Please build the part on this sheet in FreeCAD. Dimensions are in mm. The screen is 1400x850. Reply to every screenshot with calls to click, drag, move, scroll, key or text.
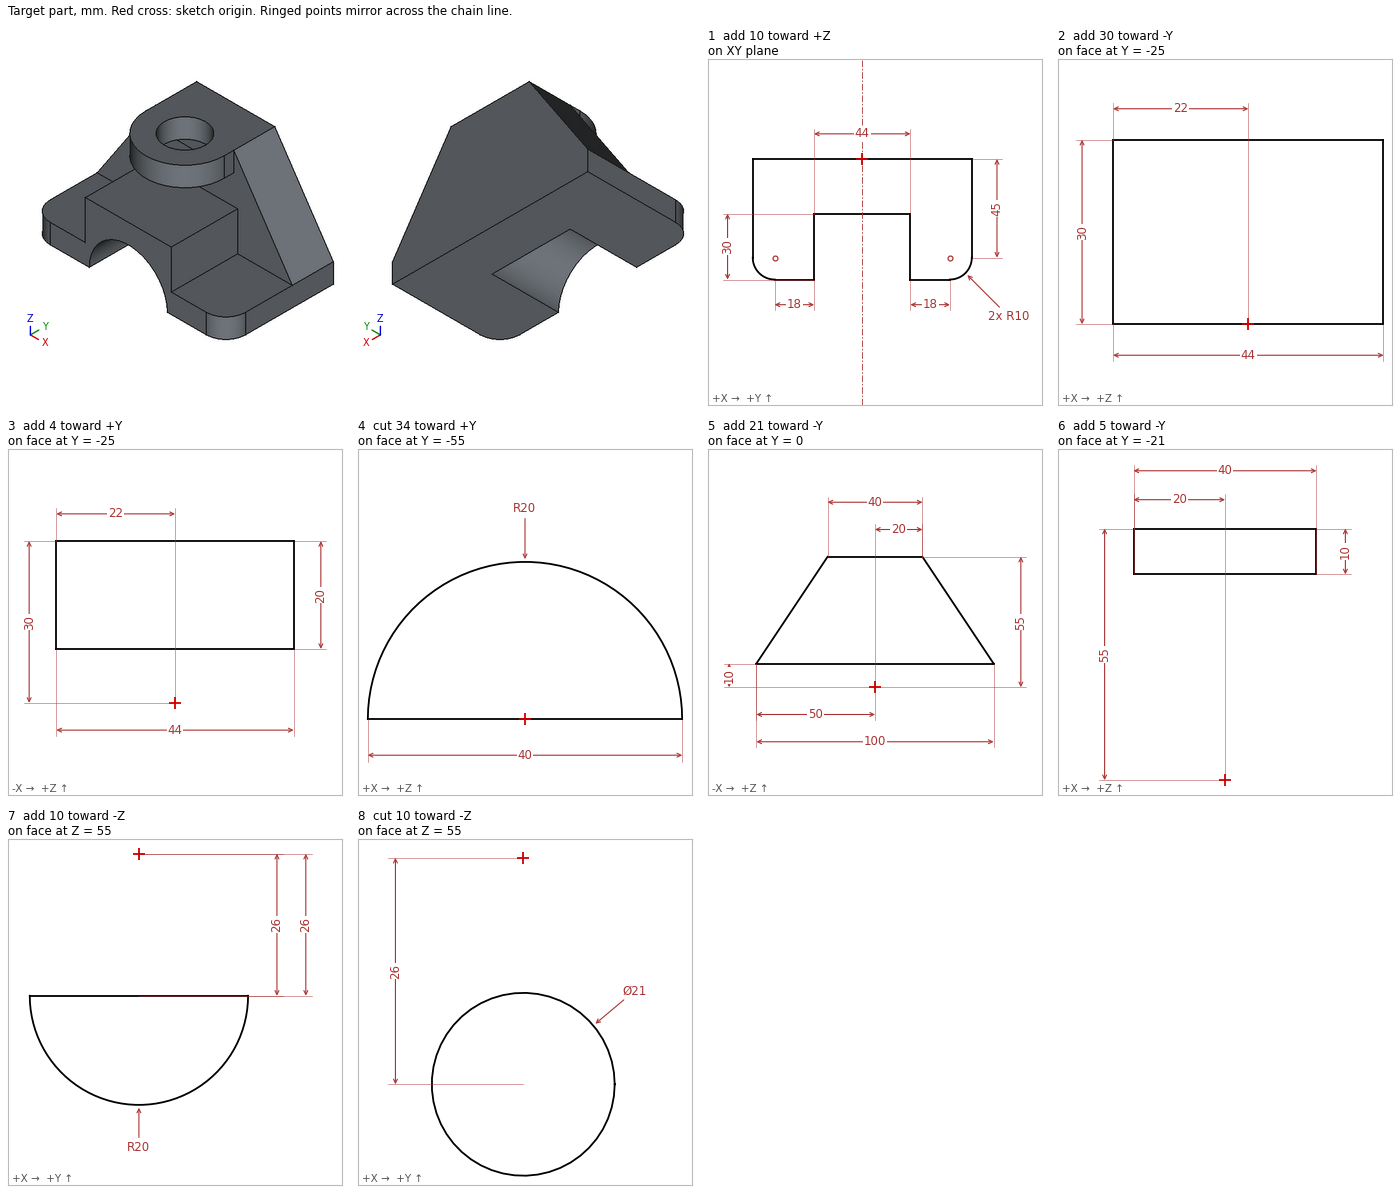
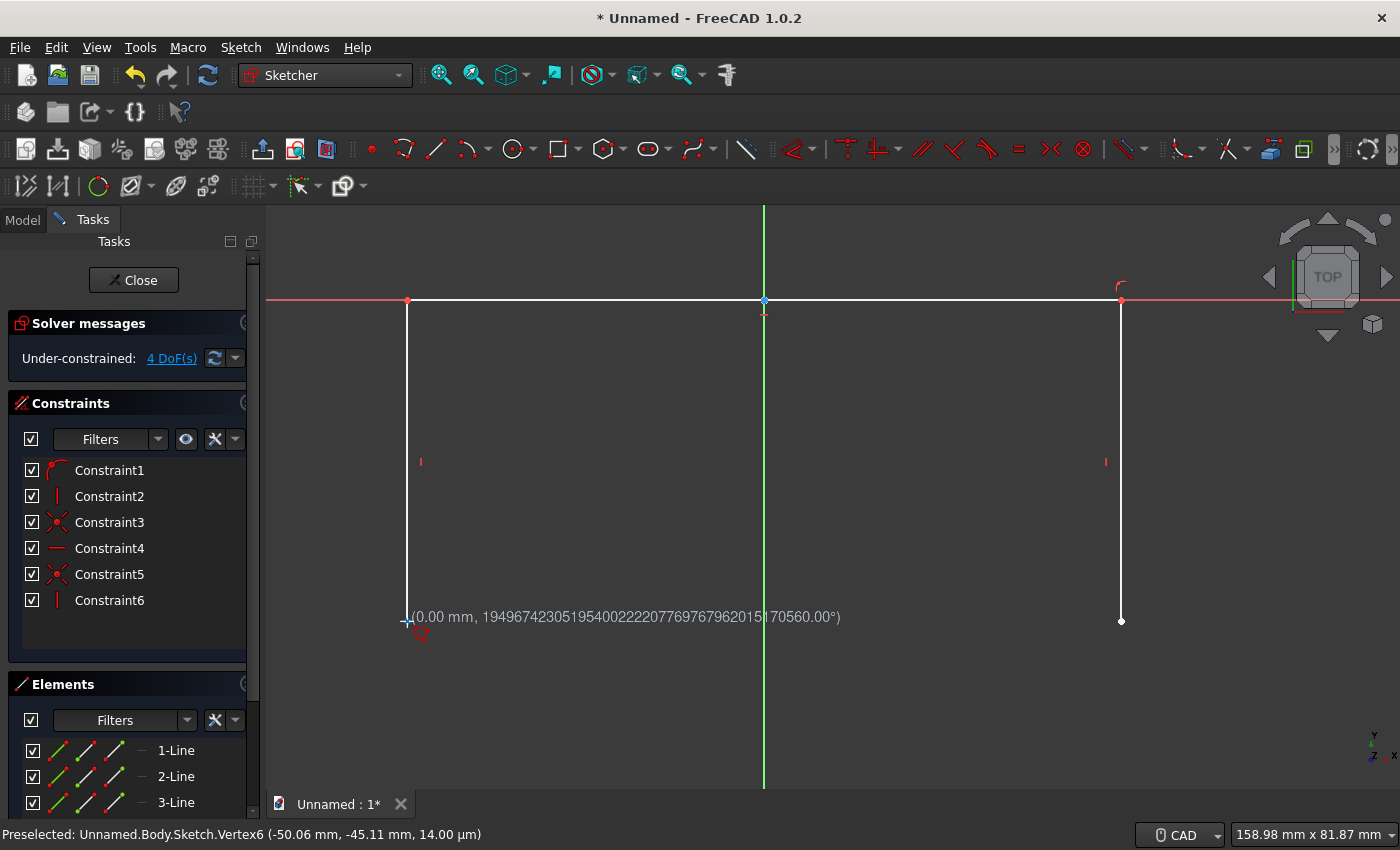
click(479, 693)
click(607, 693)
click(607, 479)
click(921, 479)
click(921, 693)
click(1049, 693)
right_click(1049, 693)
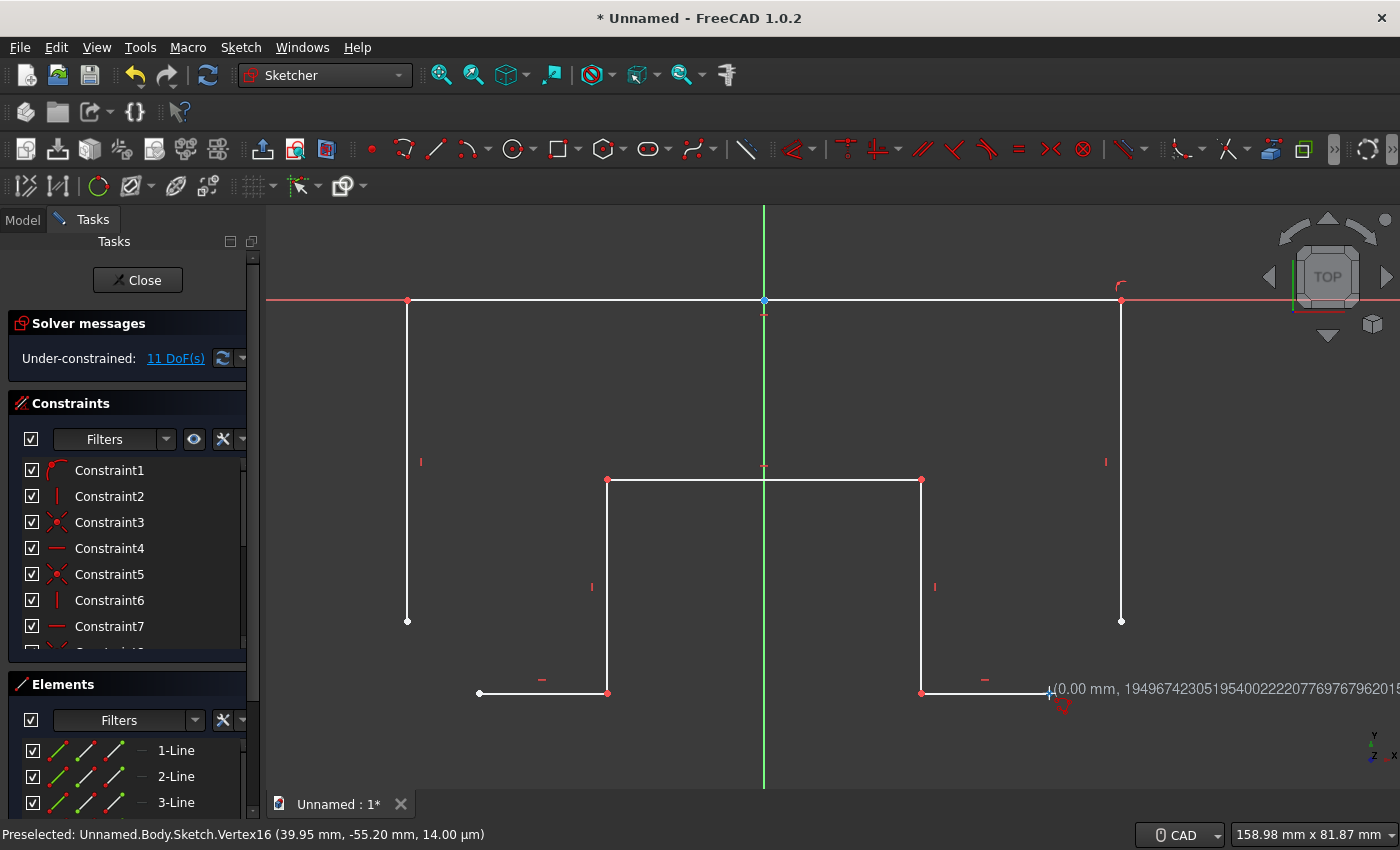
click(490, 150)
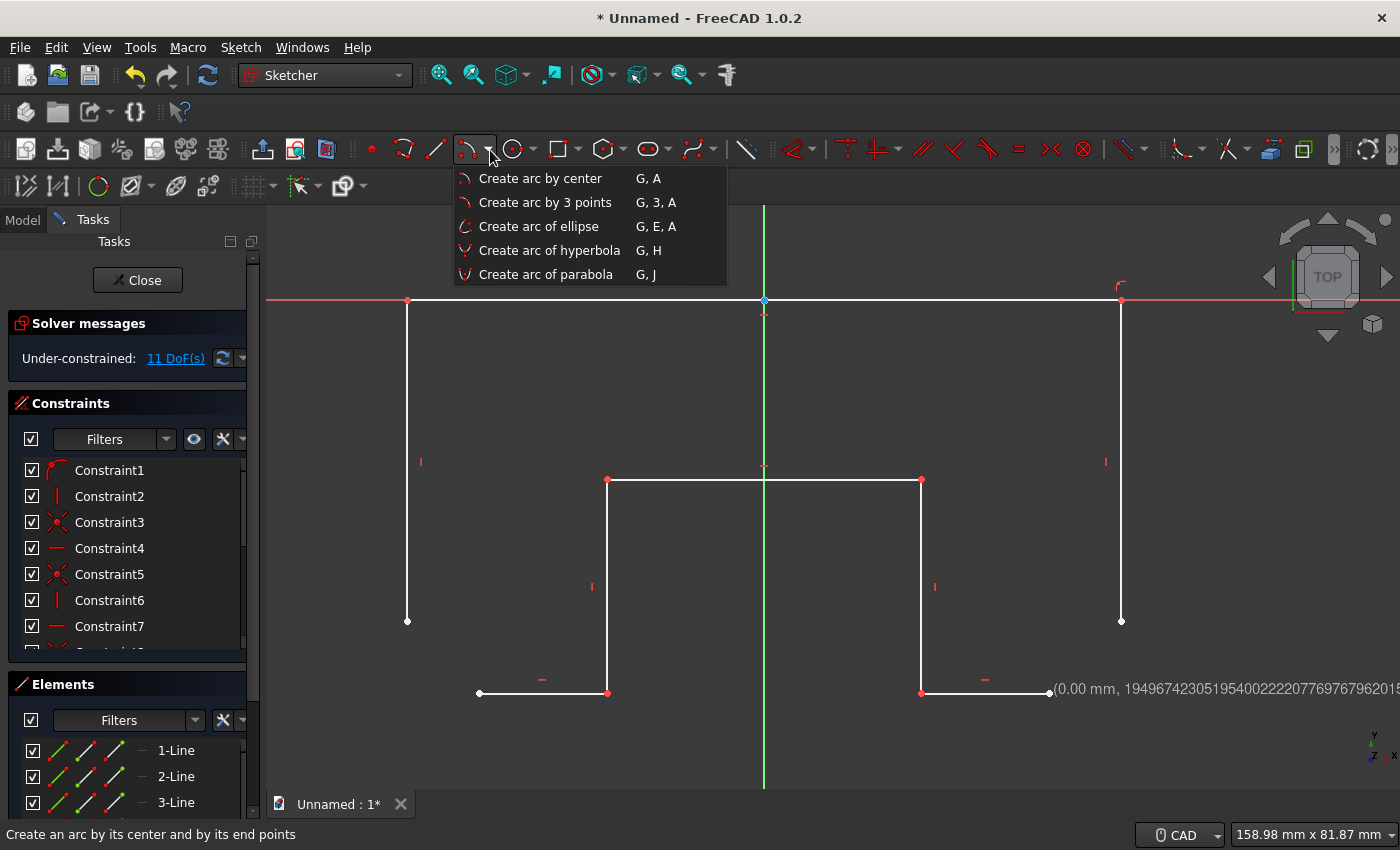
click(590, 202)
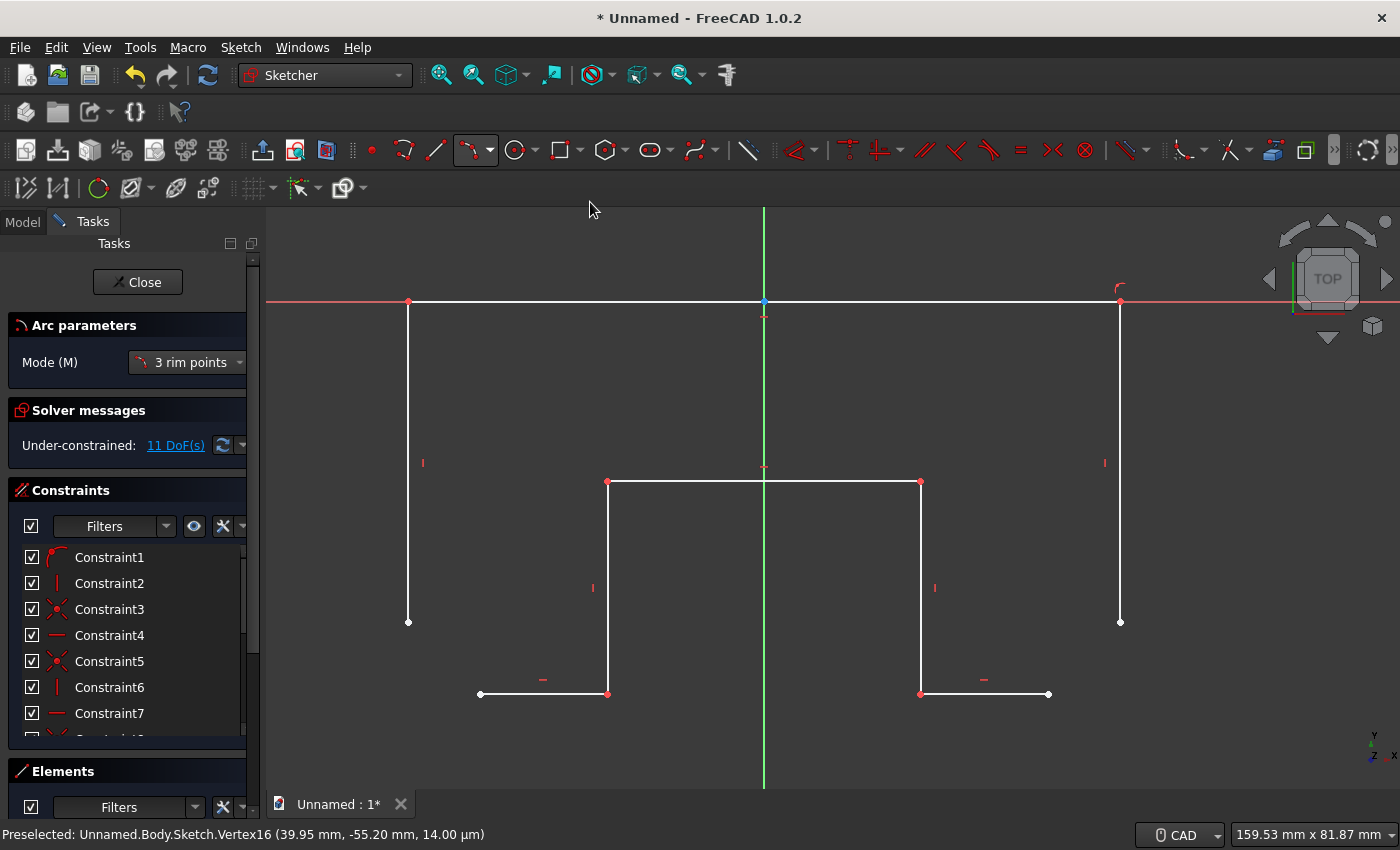
click(408, 623)
click(480, 694)
click(430, 672)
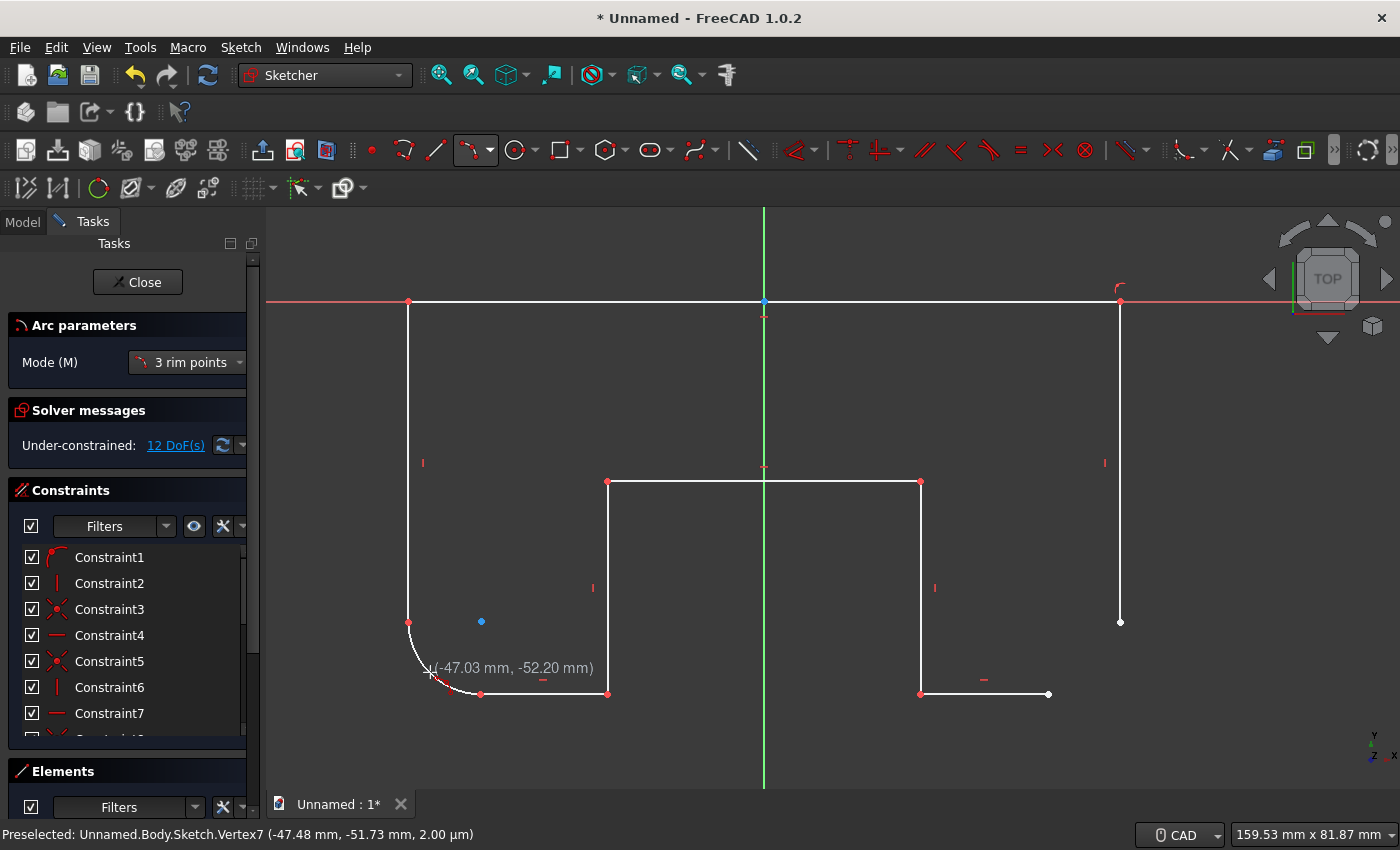
click(1048, 694)
click(1120, 623)
click(1099, 672)
key(Escape)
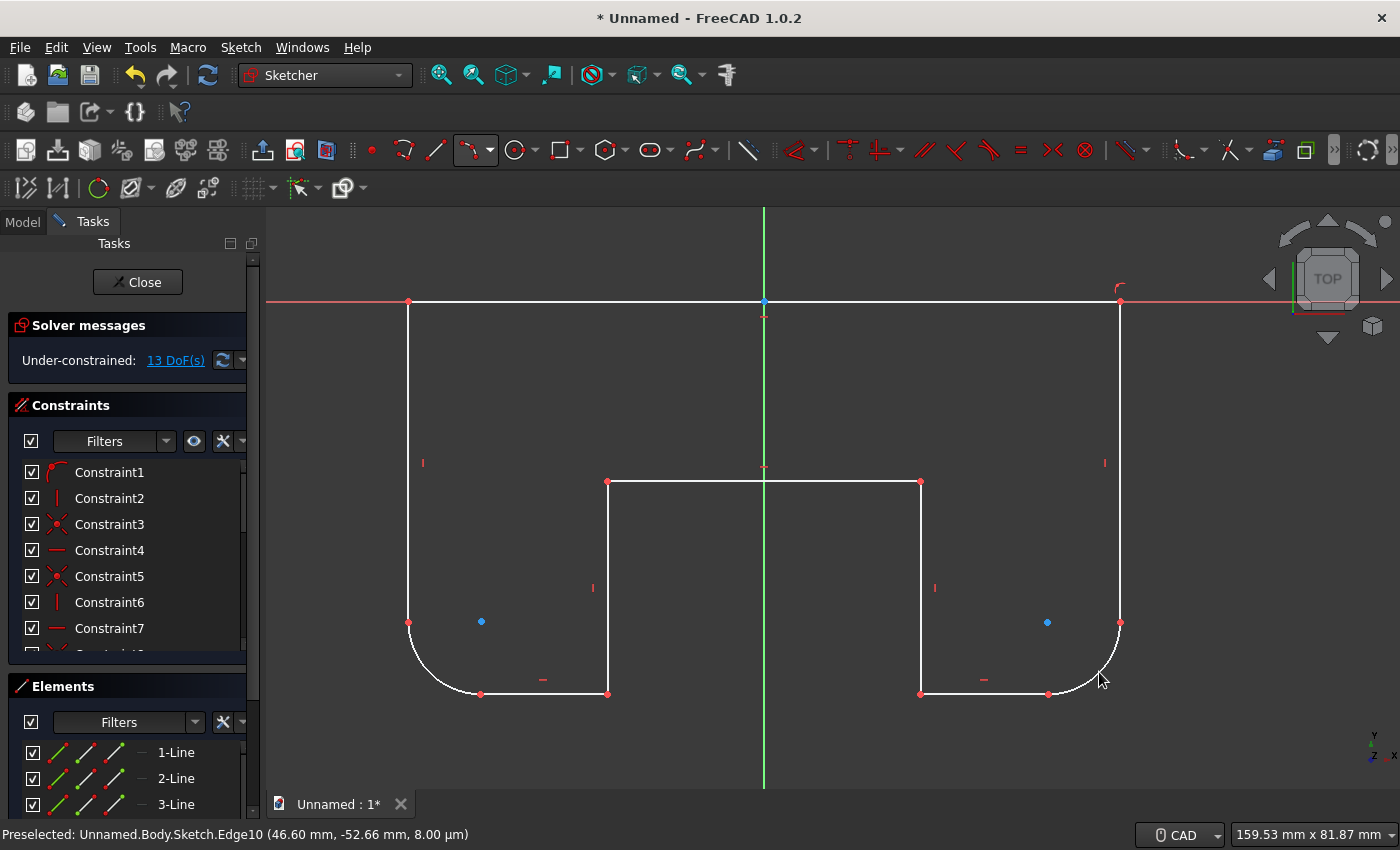
click(1120, 526)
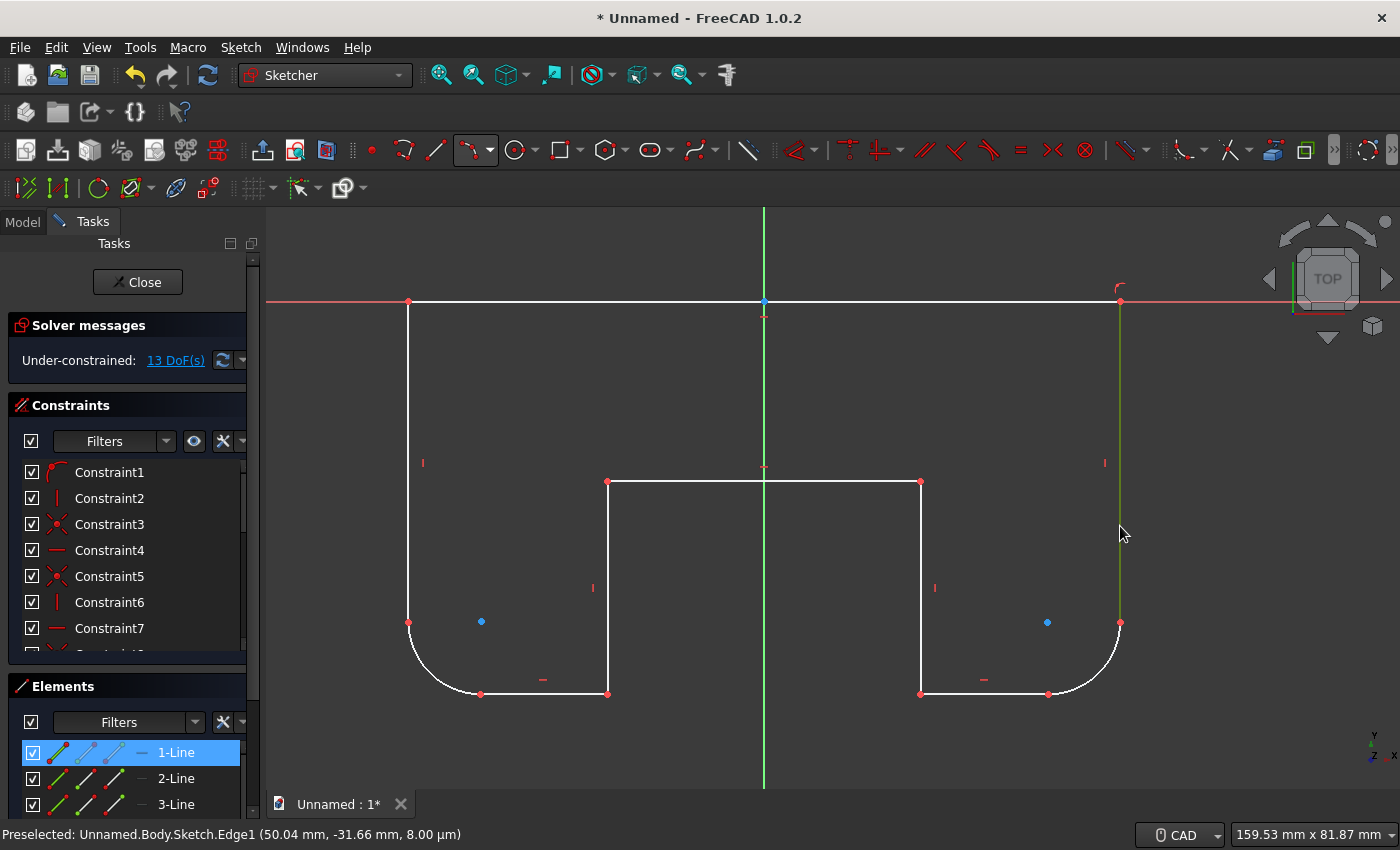
click(1081, 686)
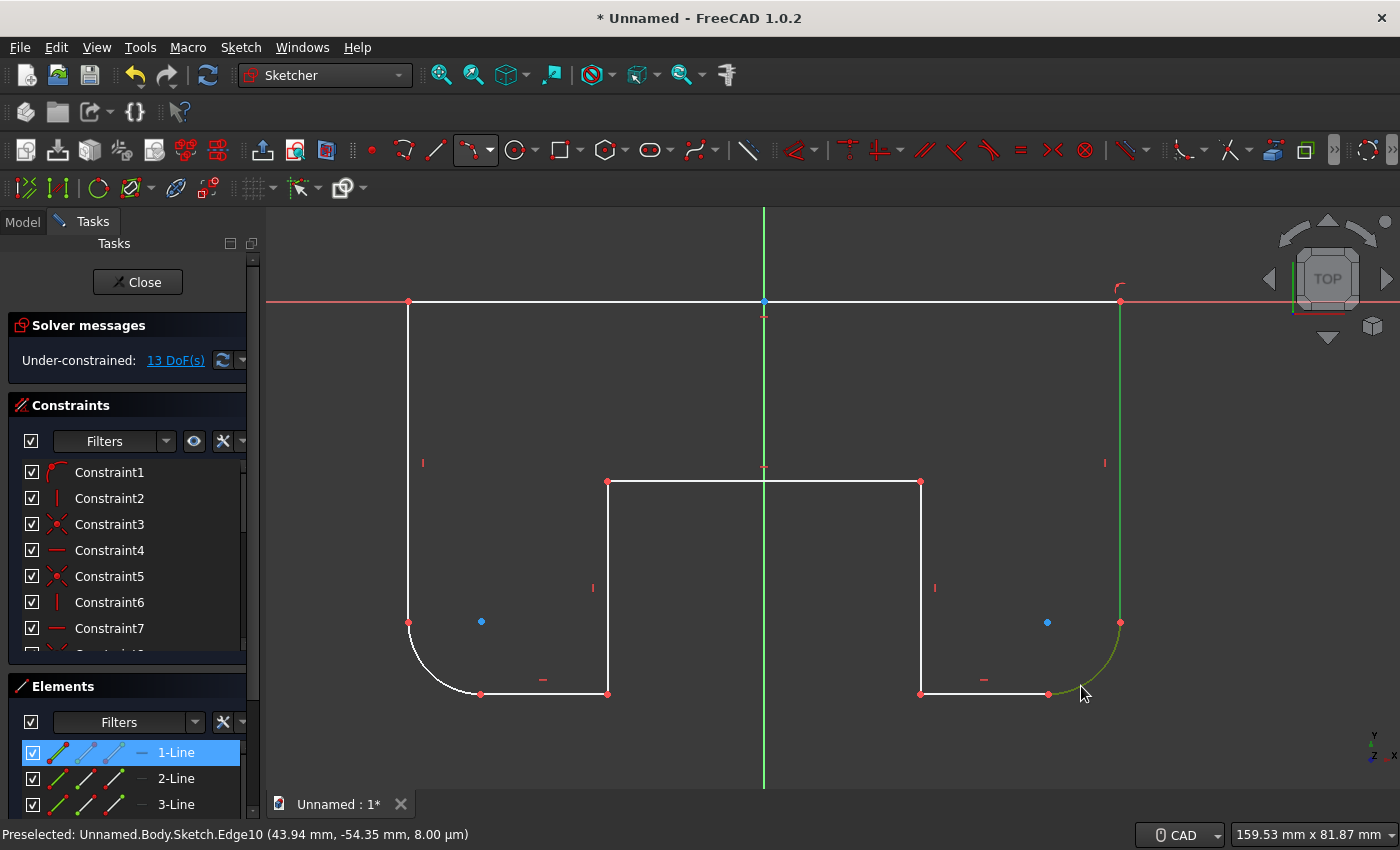
click(990, 150)